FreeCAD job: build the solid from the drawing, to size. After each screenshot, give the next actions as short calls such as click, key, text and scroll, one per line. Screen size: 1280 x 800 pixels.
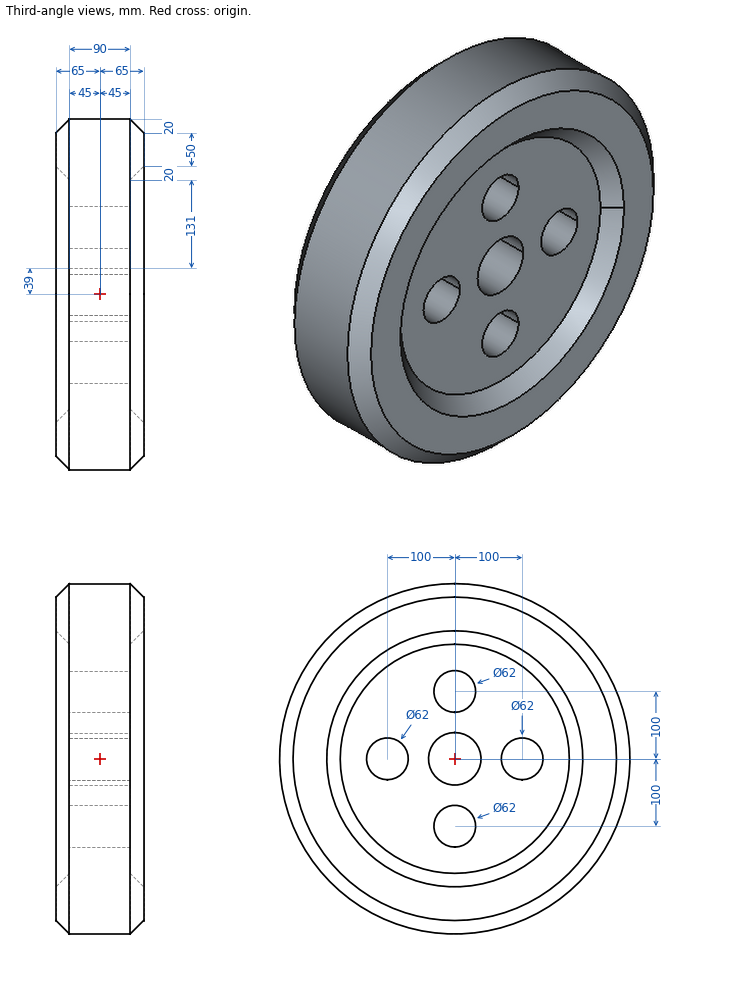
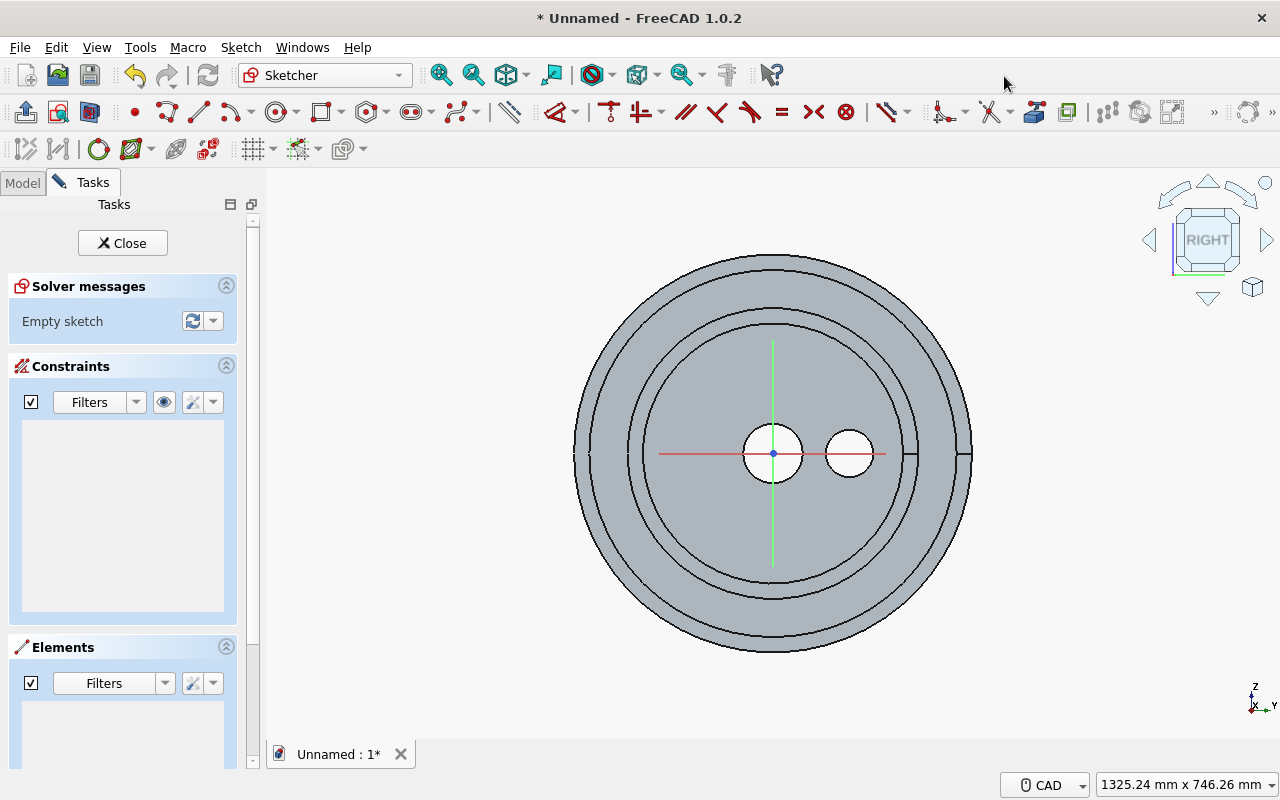
scroll(803, 525, up, 6)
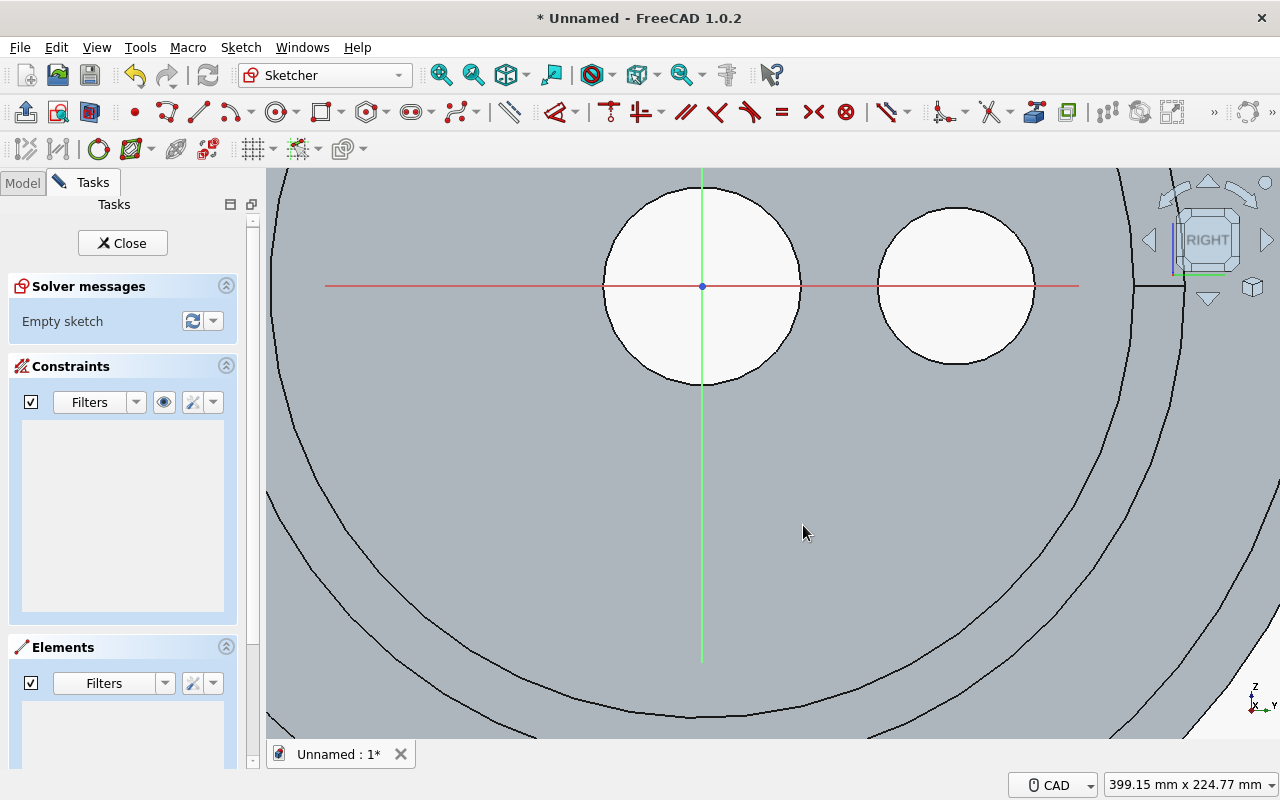
key(g)
key(c)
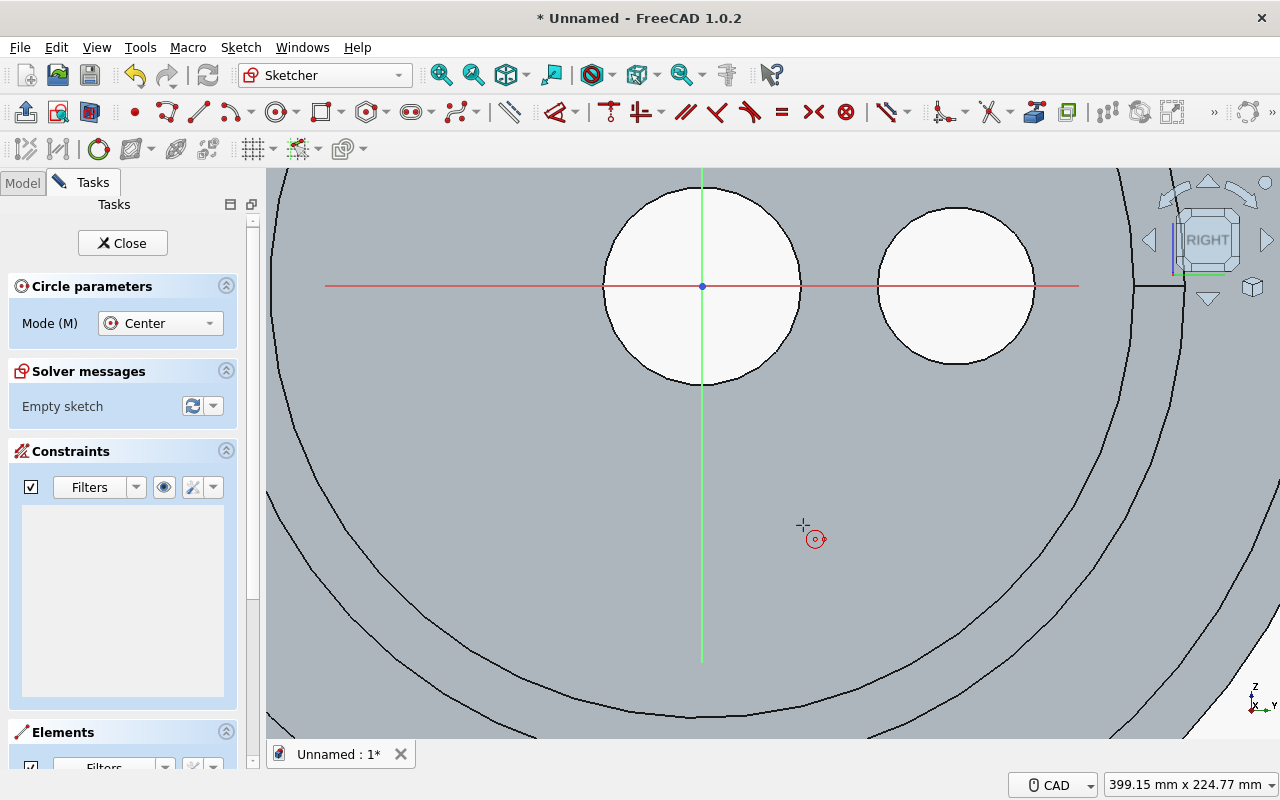
click(702, 540)
click(758, 485)
key(Escape)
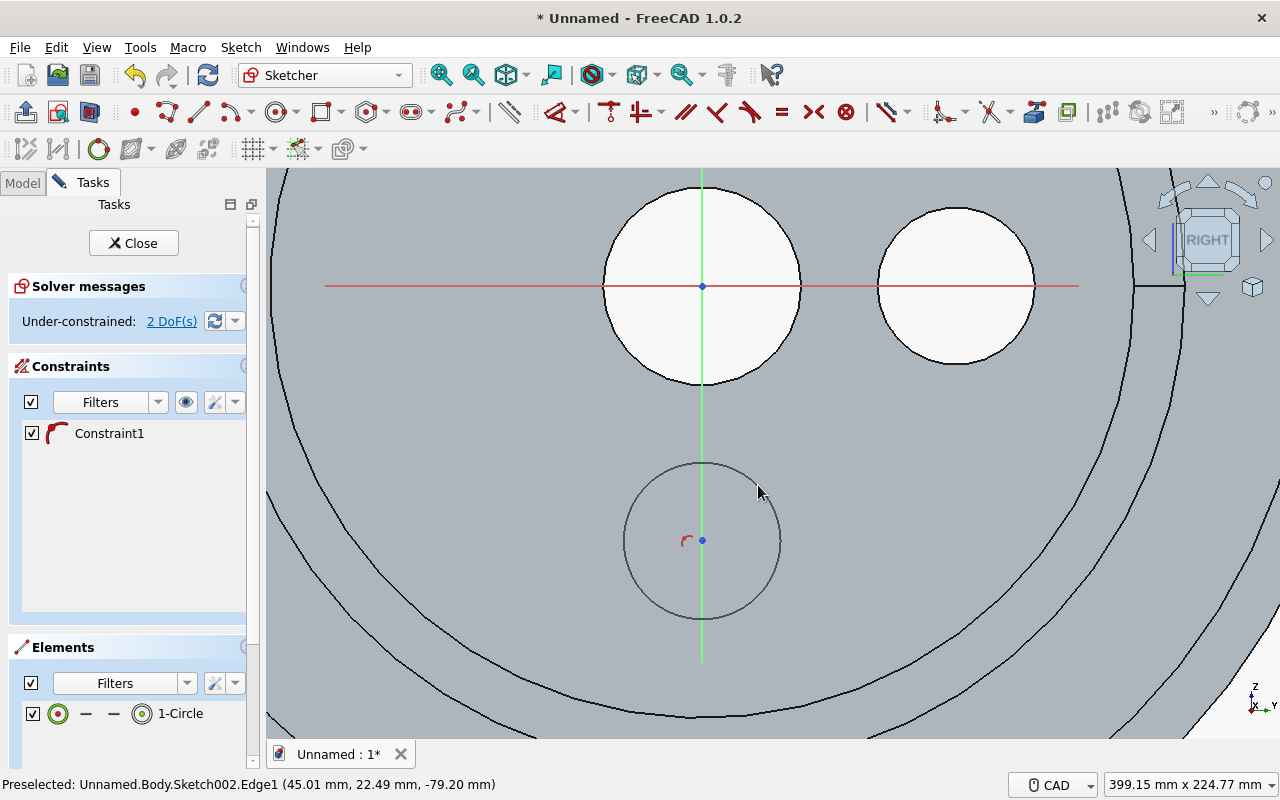
key(d)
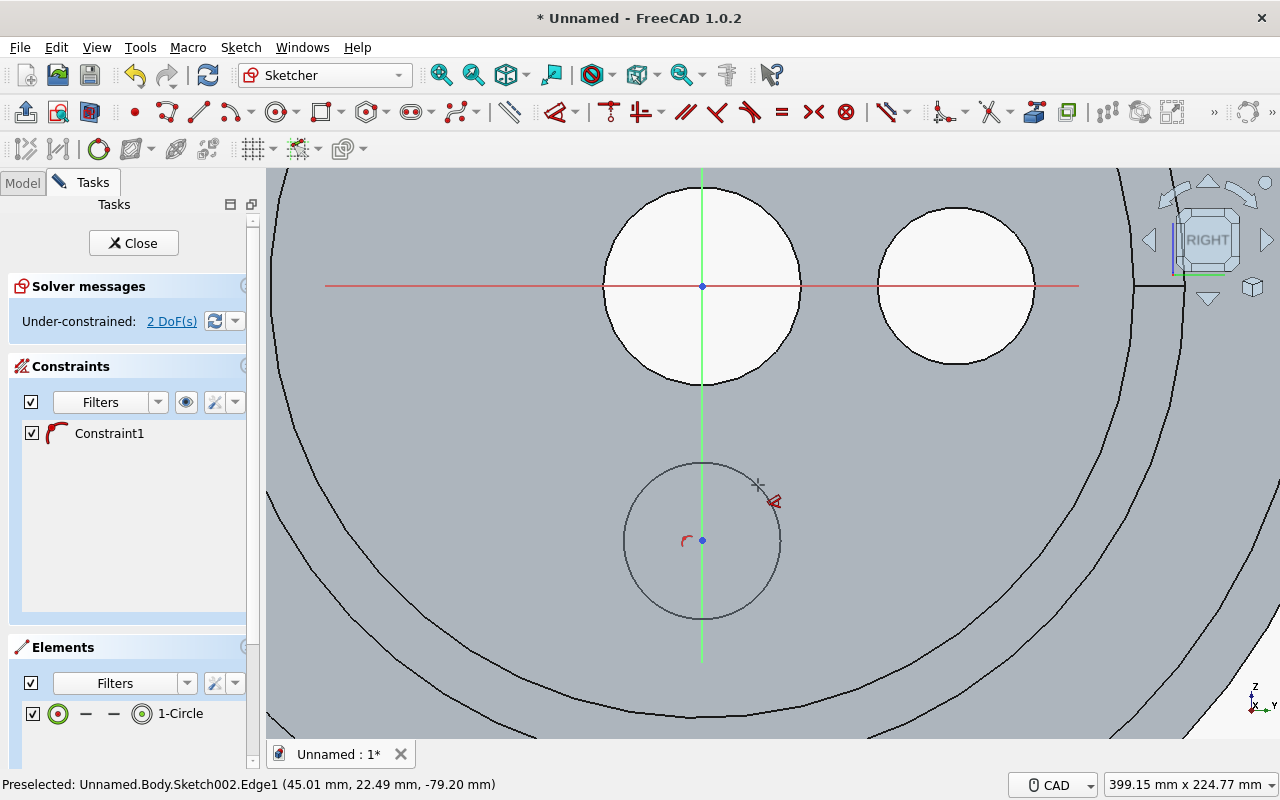
click(757, 485)
click(779, 462)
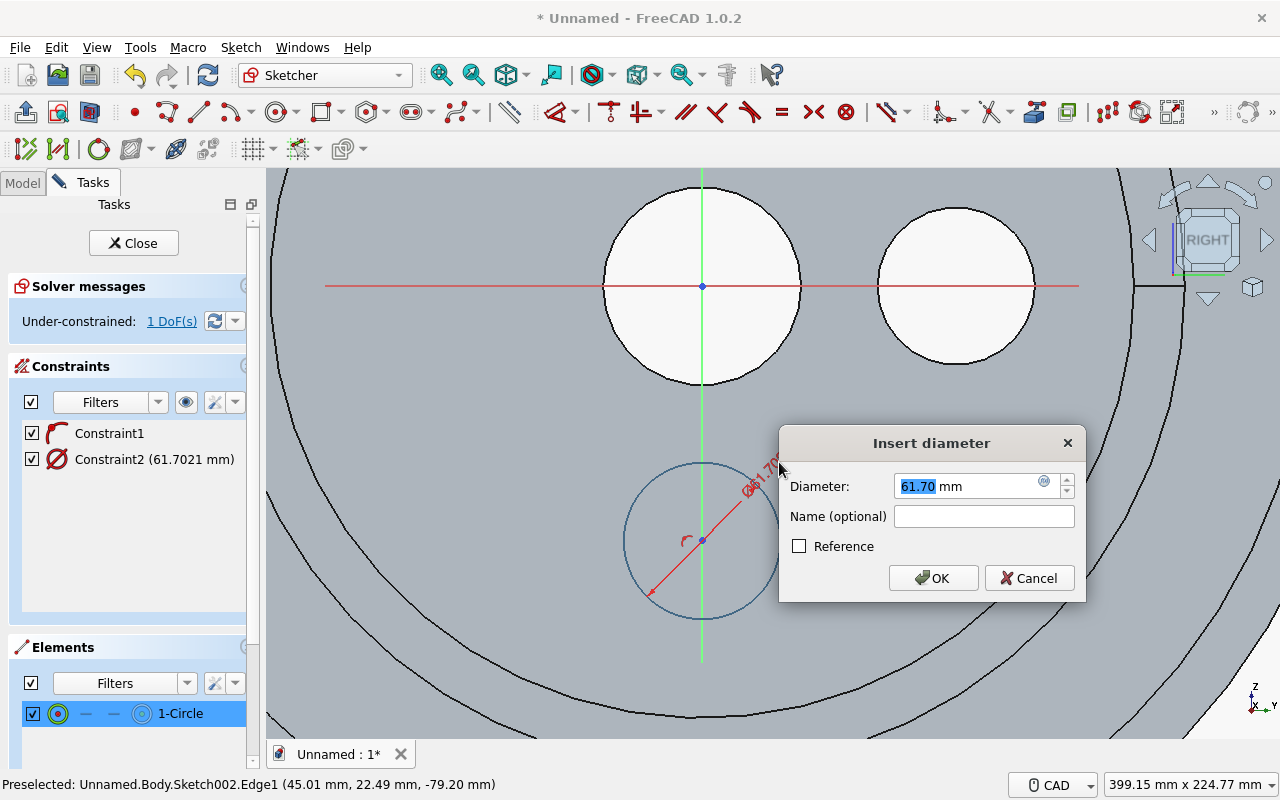
text(62)
key(Return)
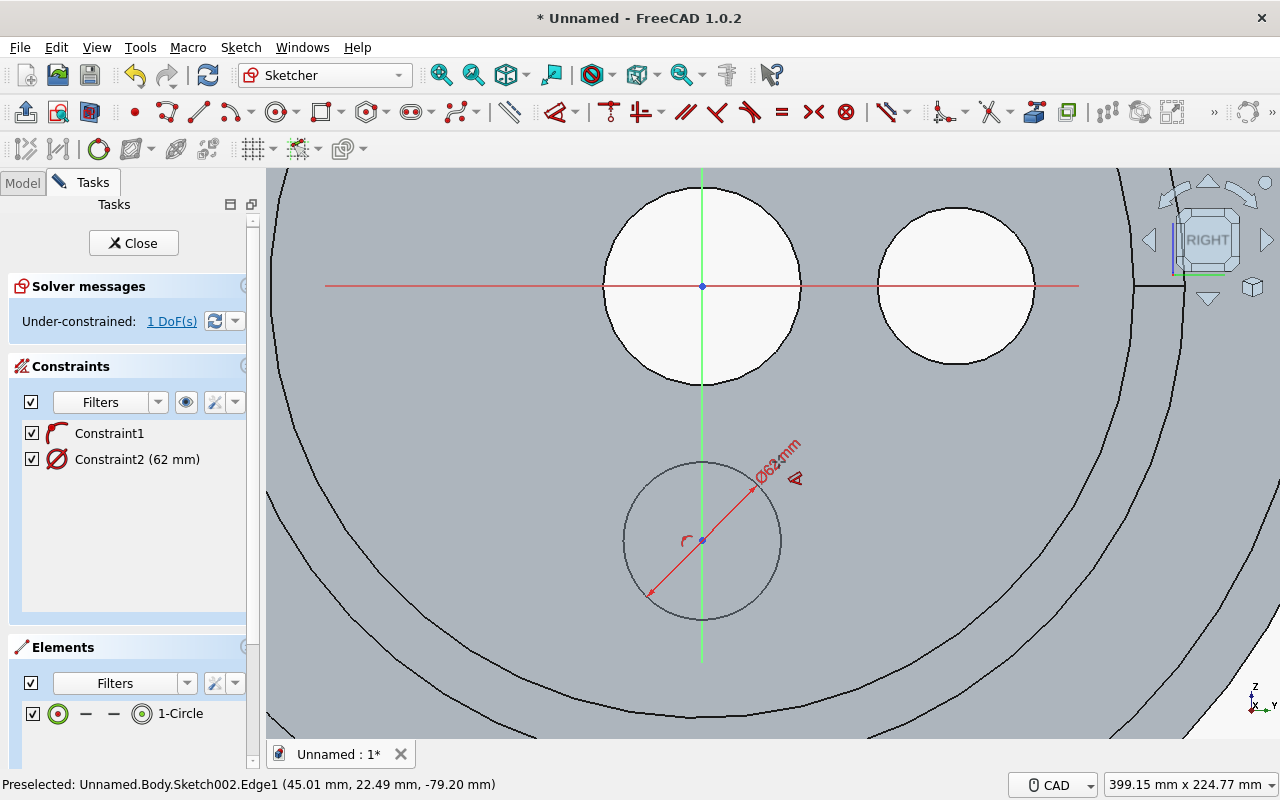
click(702, 541)
click(736, 414)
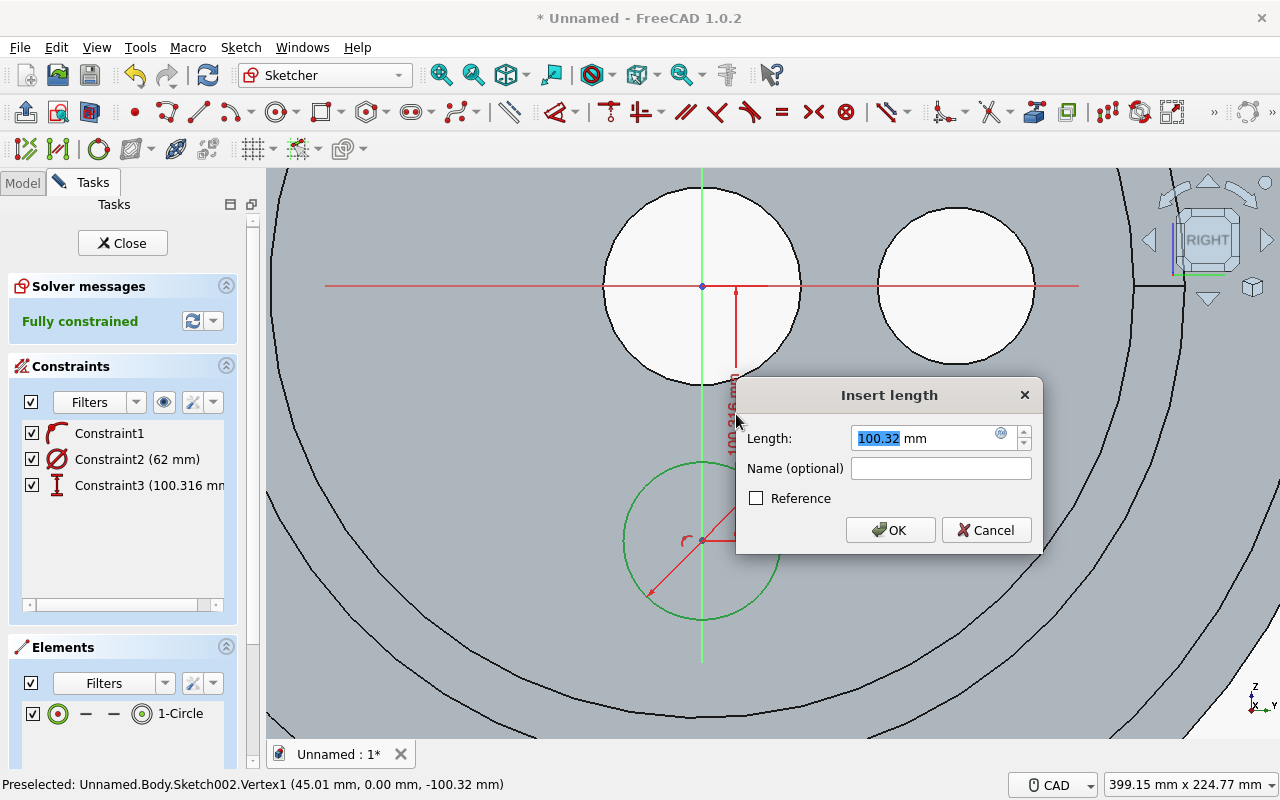
text(100)
key(Return)
key(Escape)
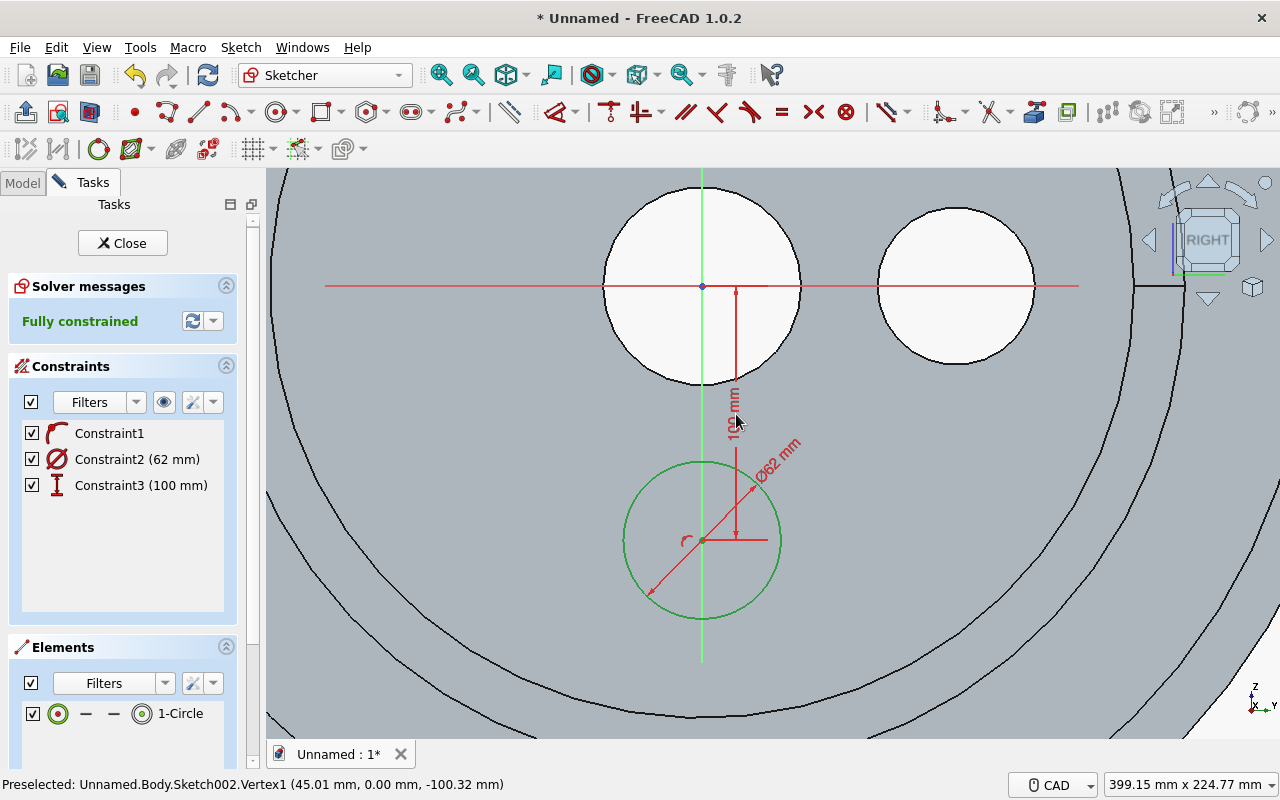
click(123, 243)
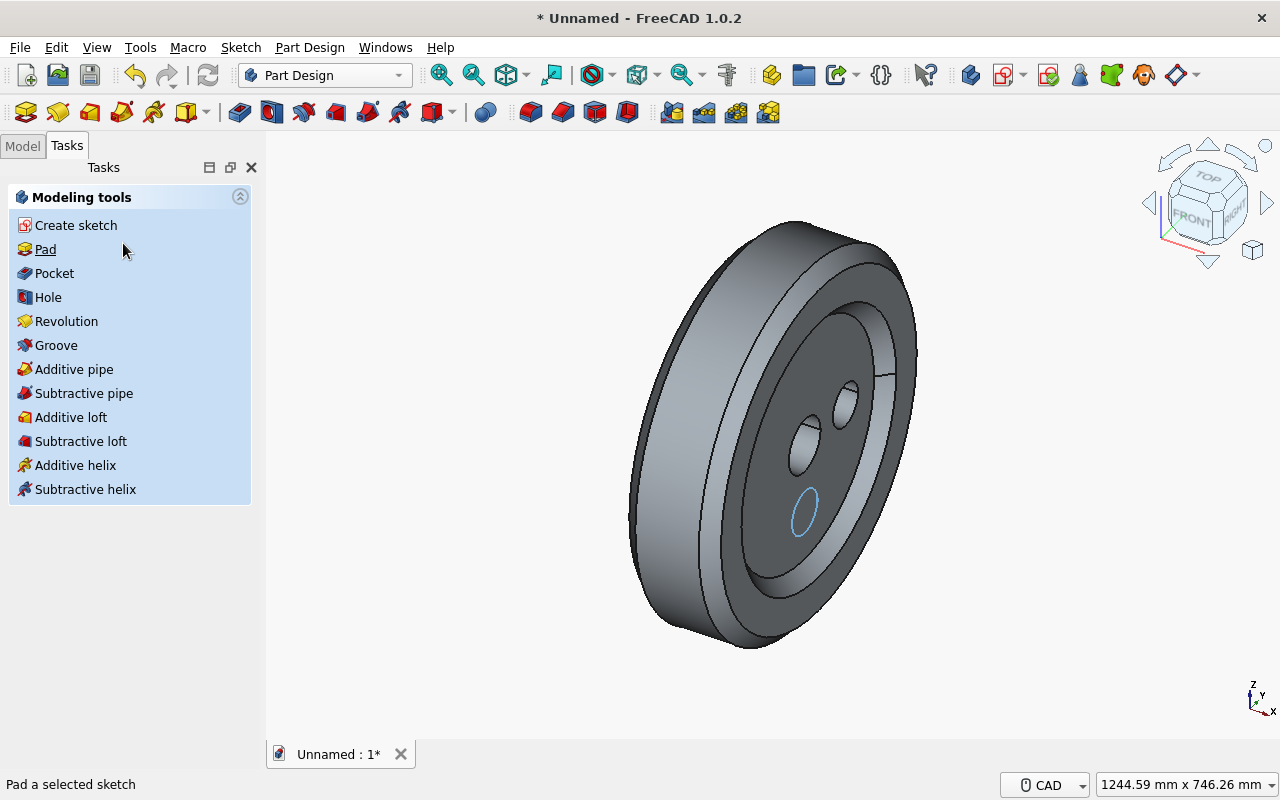
click(240, 112)